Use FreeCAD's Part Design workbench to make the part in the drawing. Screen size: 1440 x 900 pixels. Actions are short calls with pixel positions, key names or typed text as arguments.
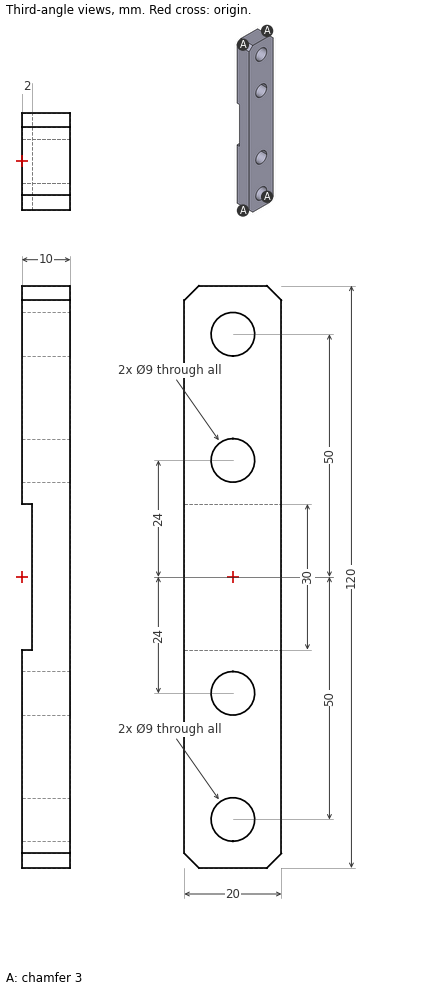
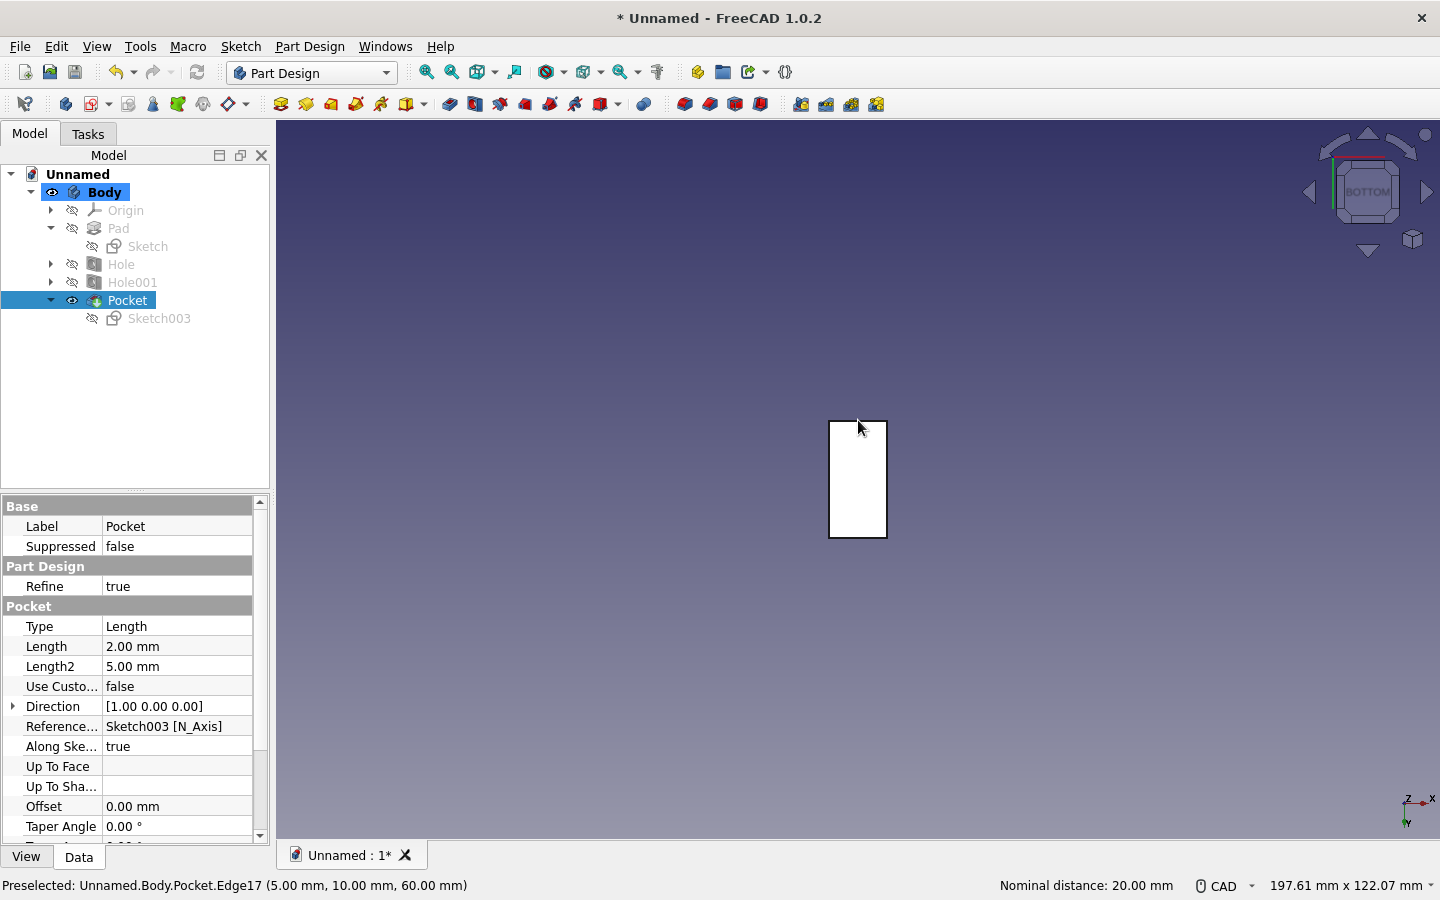
click(858, 420, ctrl)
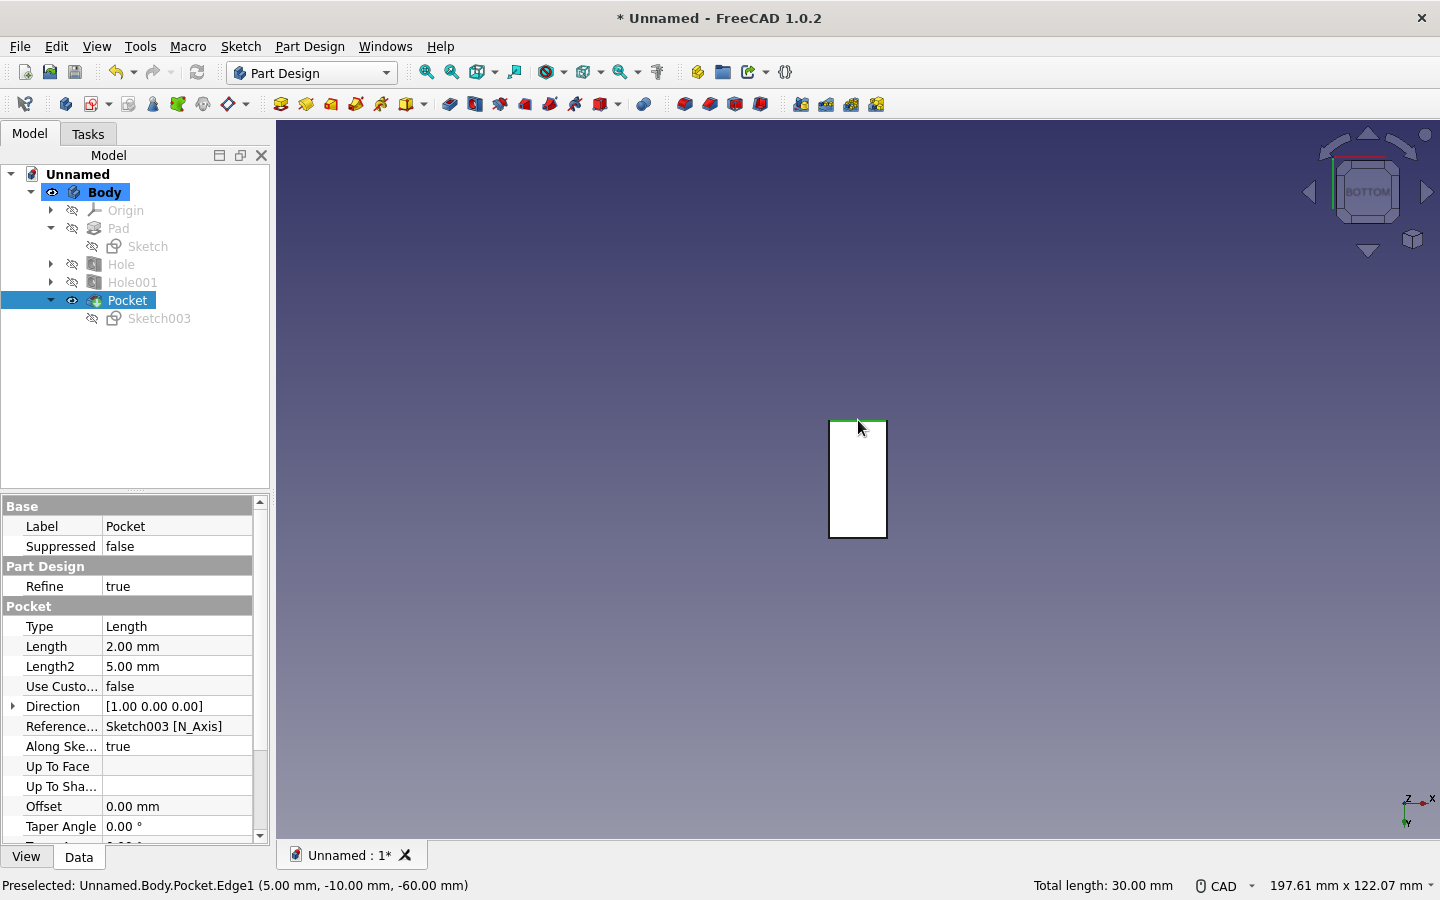
click(858, 537, ctrl)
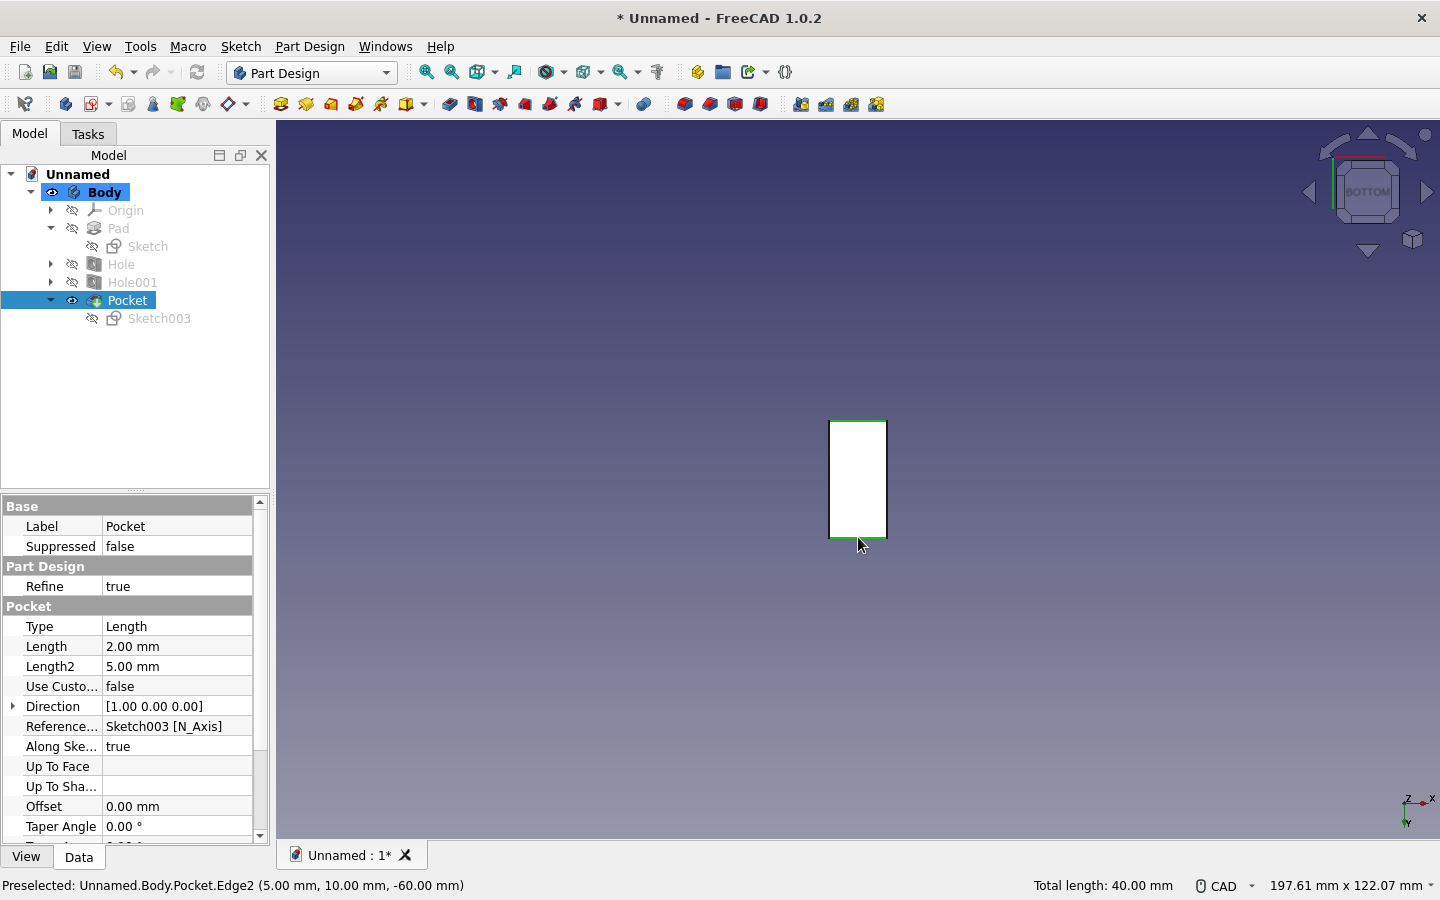
click(710, 104)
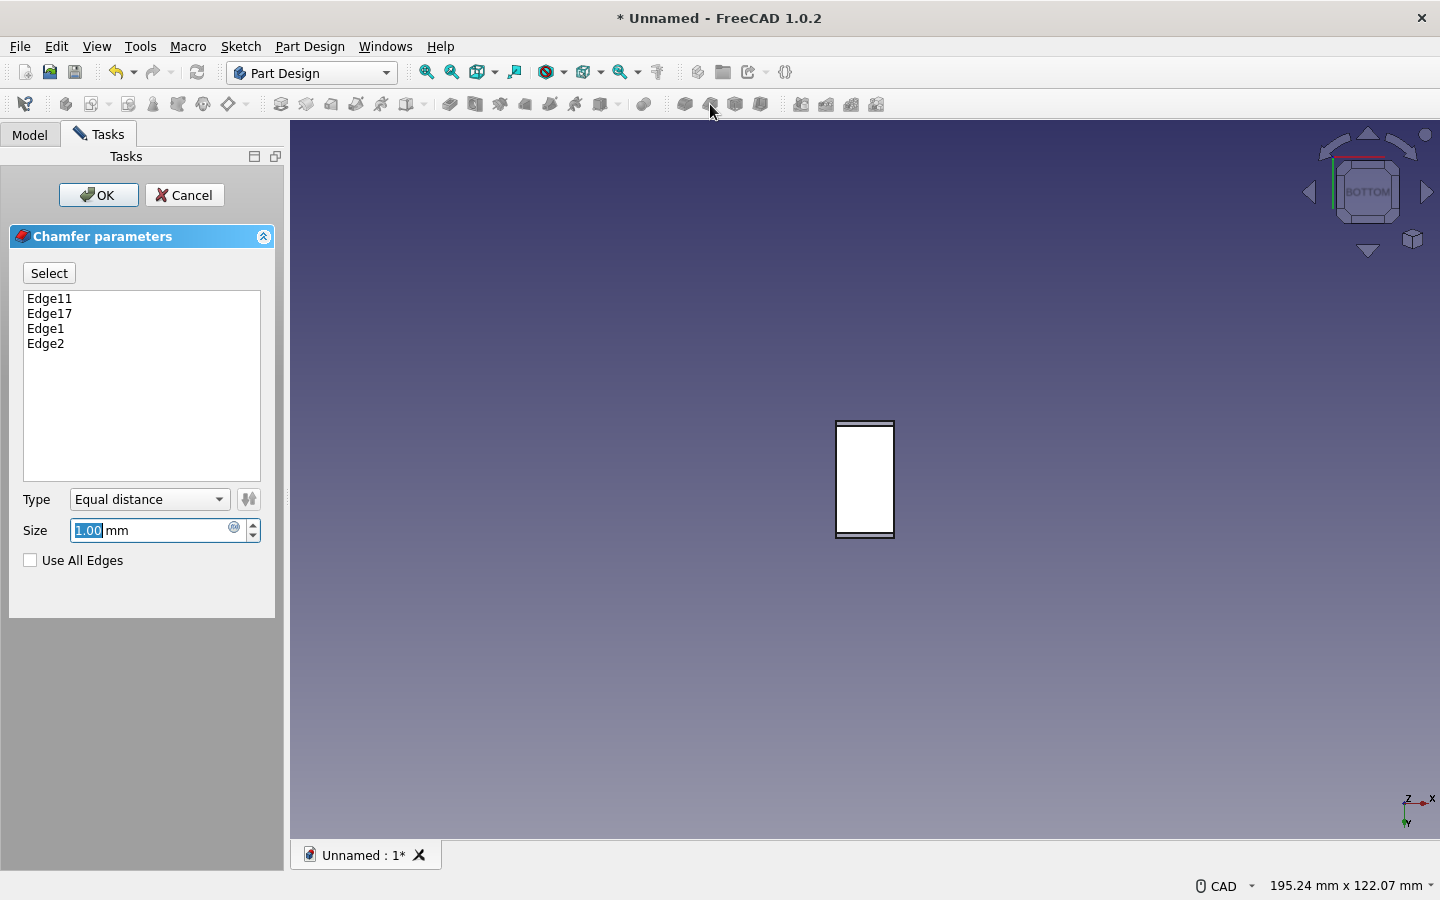
text(3)
key(Tab)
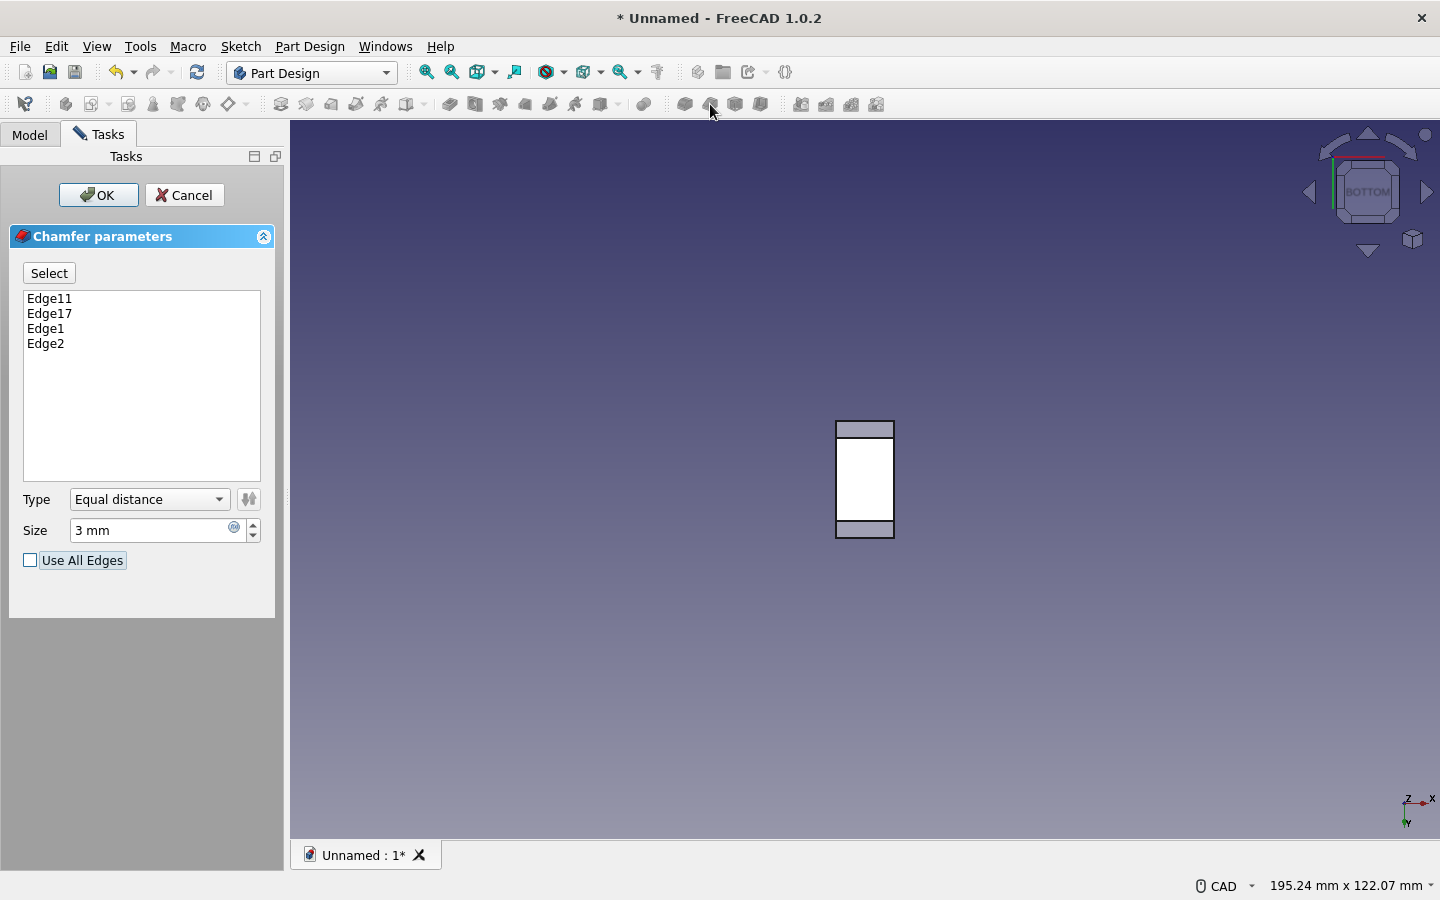
click(99, 195)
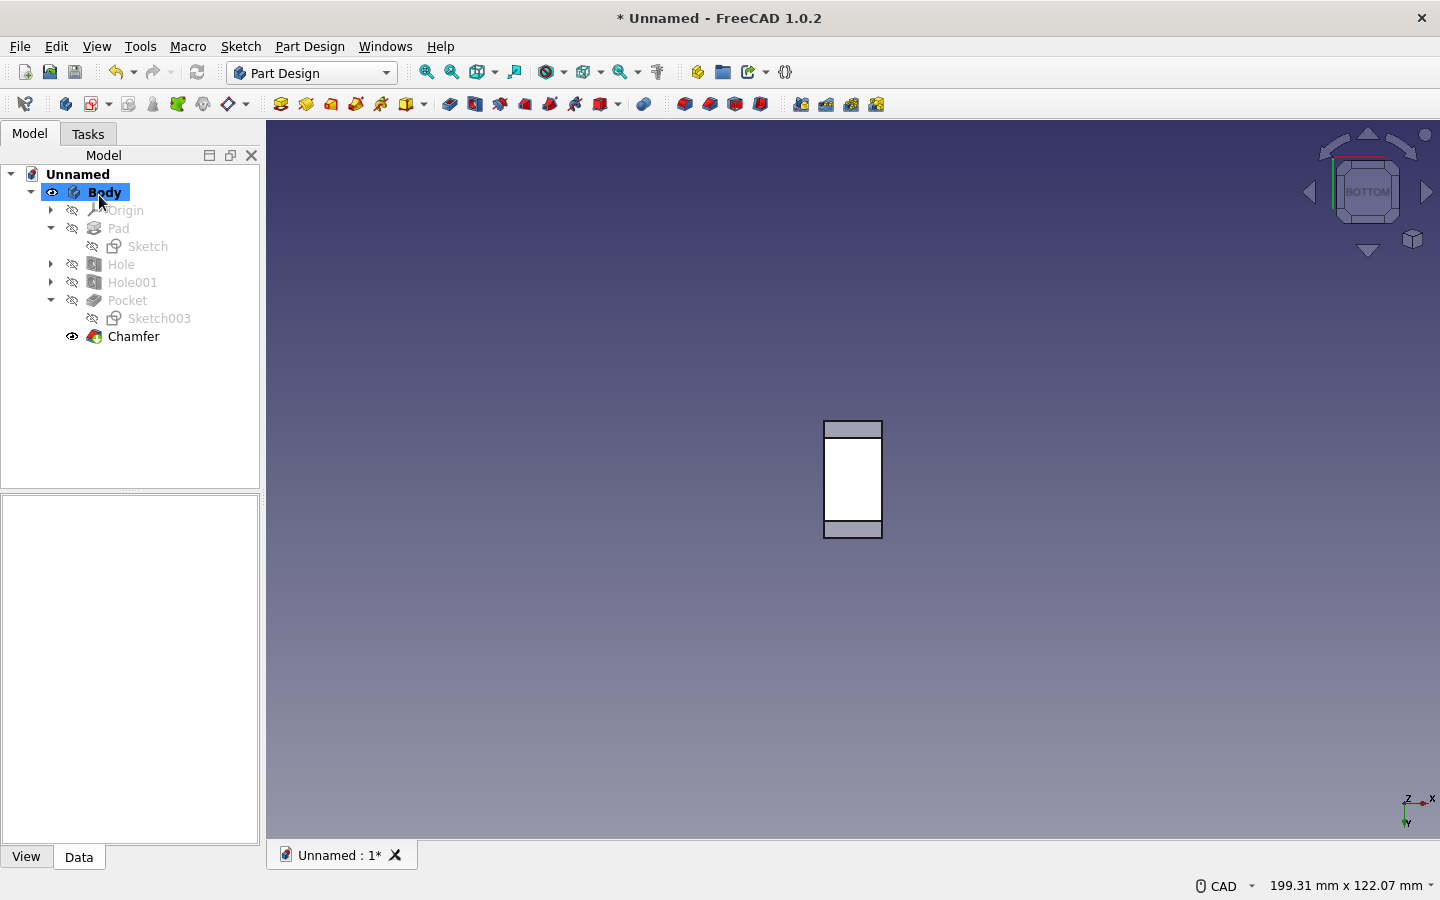
key(0)